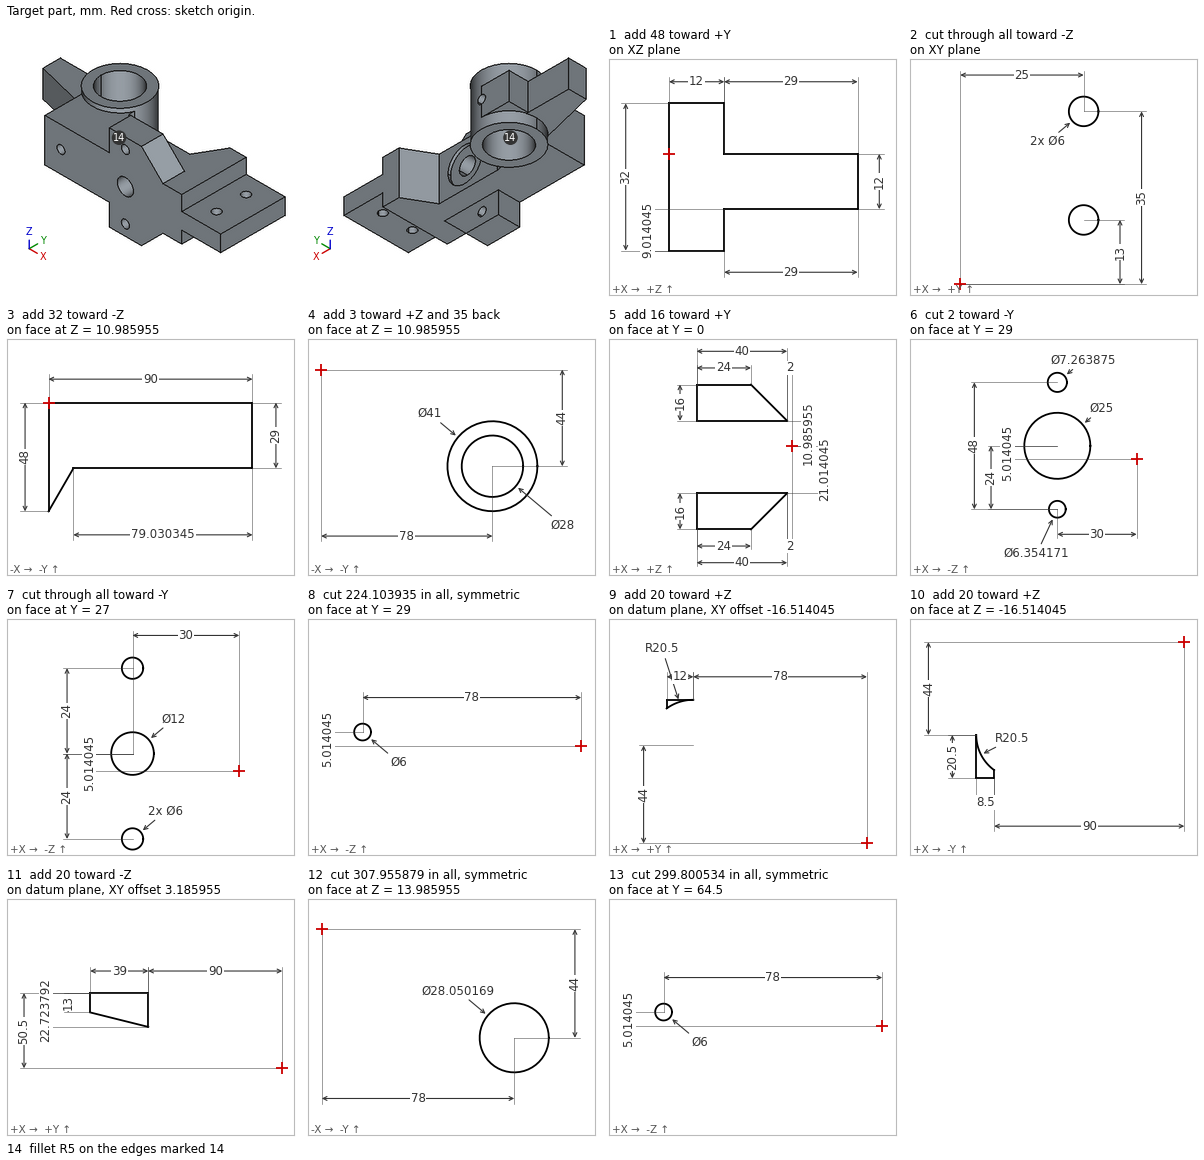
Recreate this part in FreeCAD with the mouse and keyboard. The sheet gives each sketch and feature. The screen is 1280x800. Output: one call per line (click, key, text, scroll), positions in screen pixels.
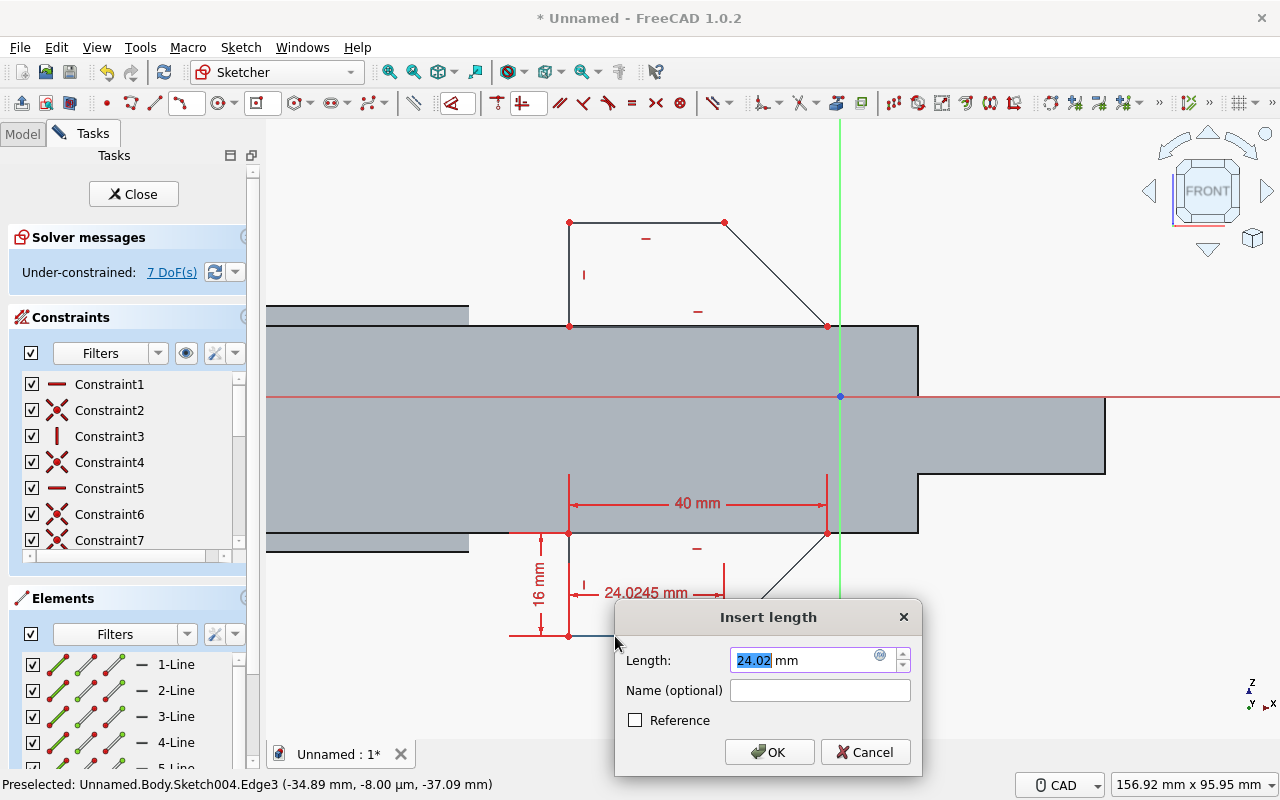
text(24)
key(Return)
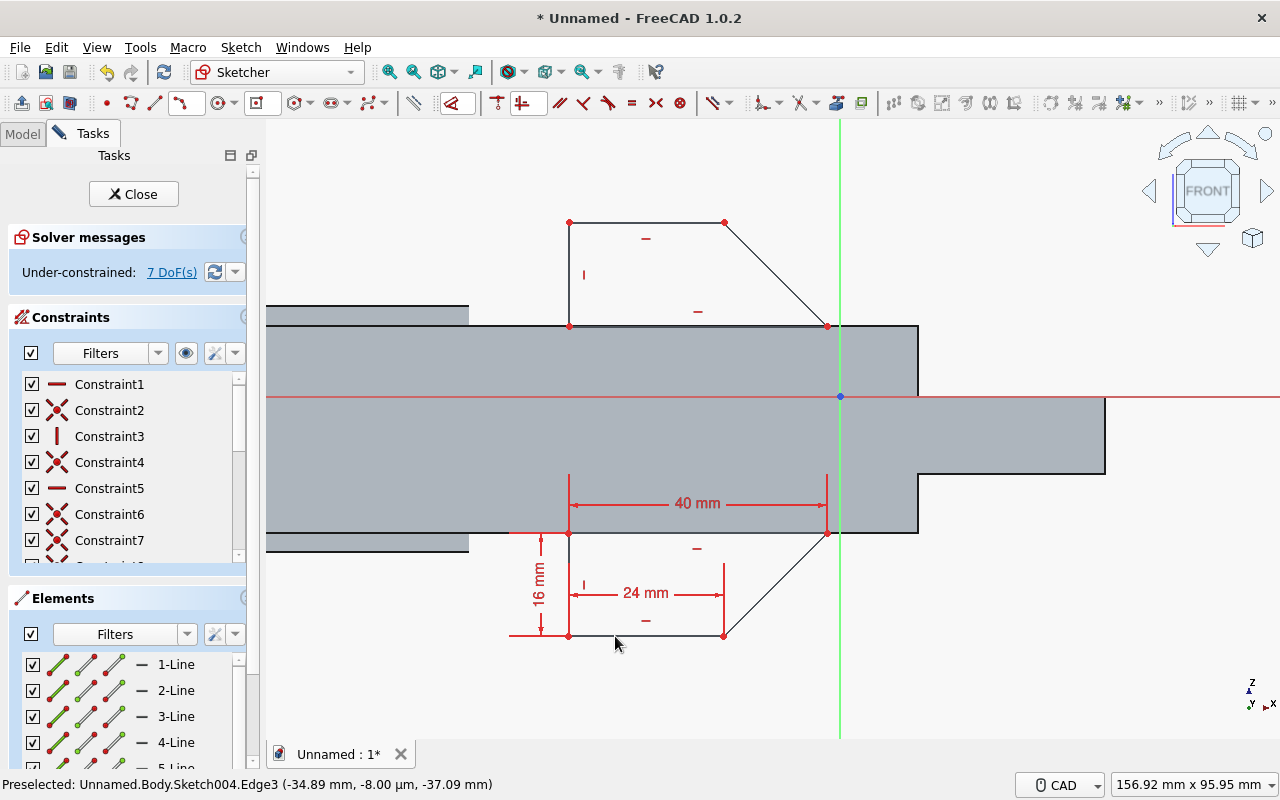
click(677, 223)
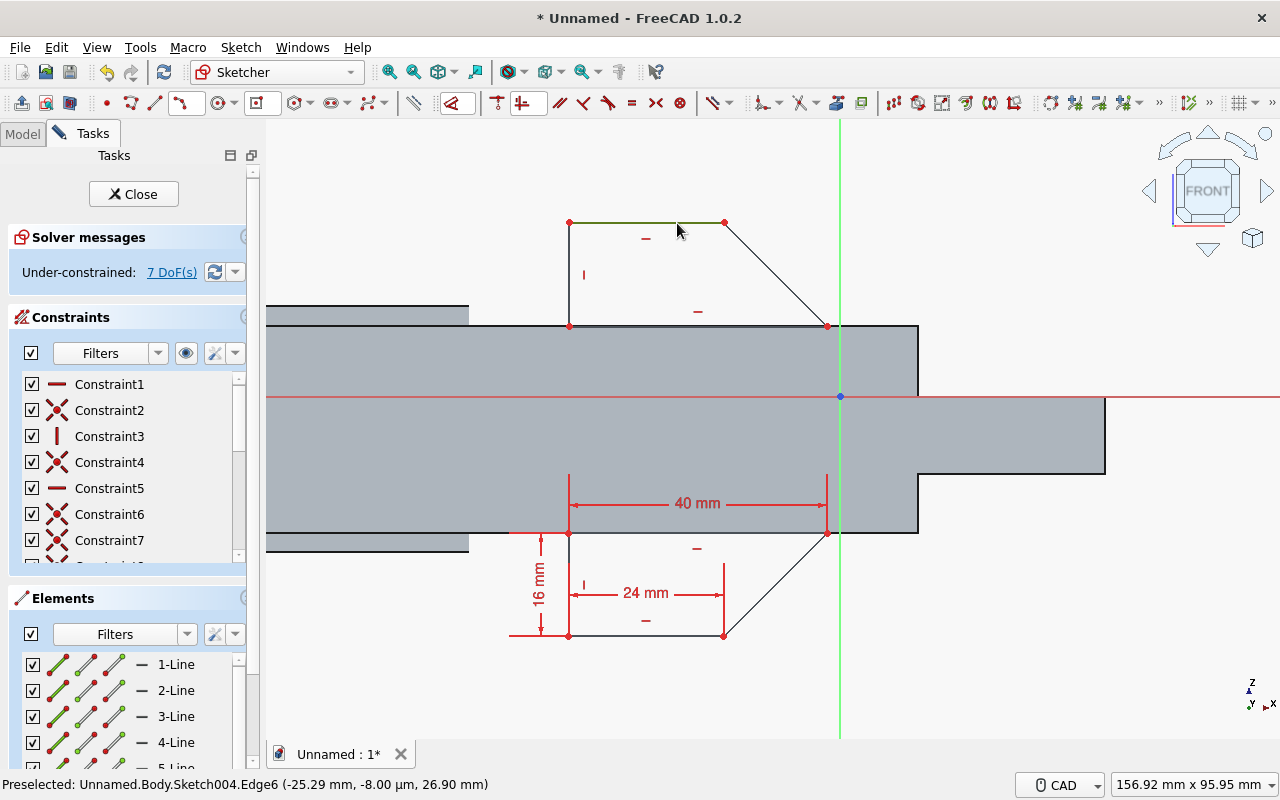
key(l)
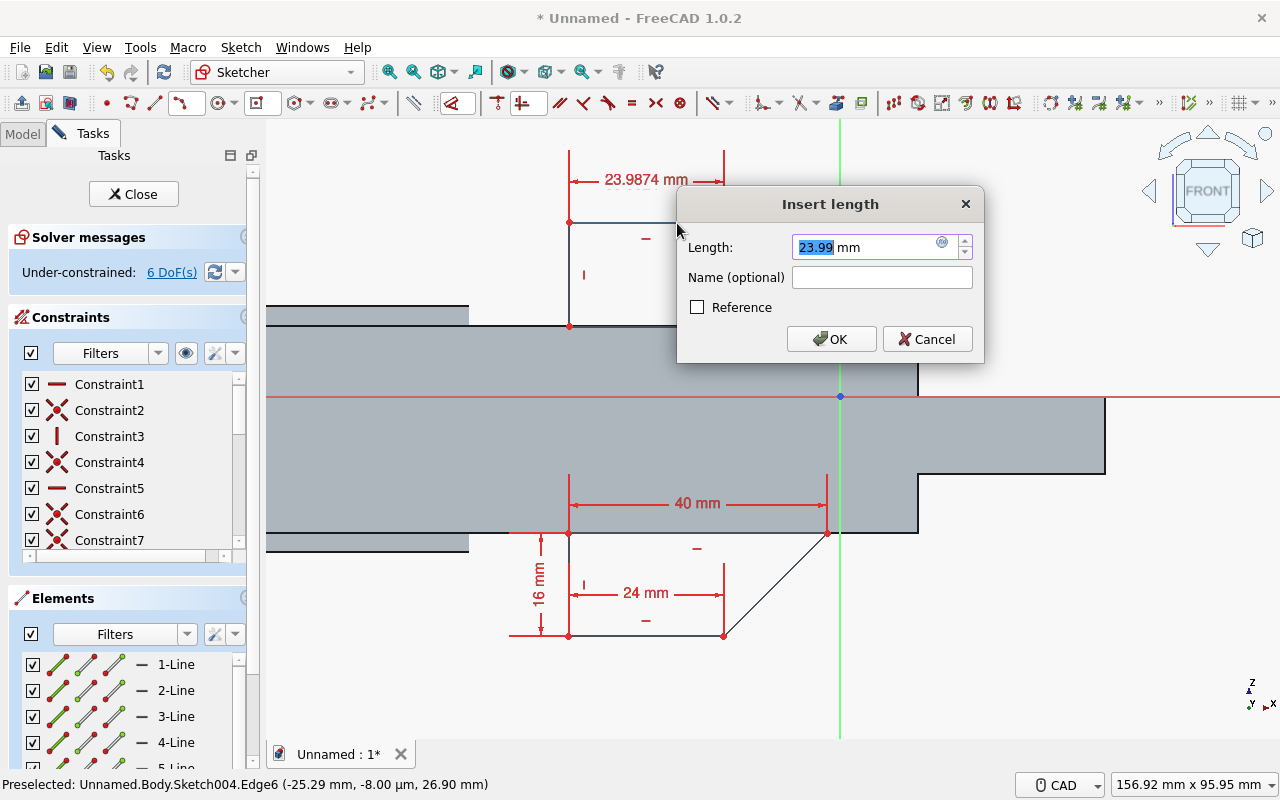
text(24)
key(Return)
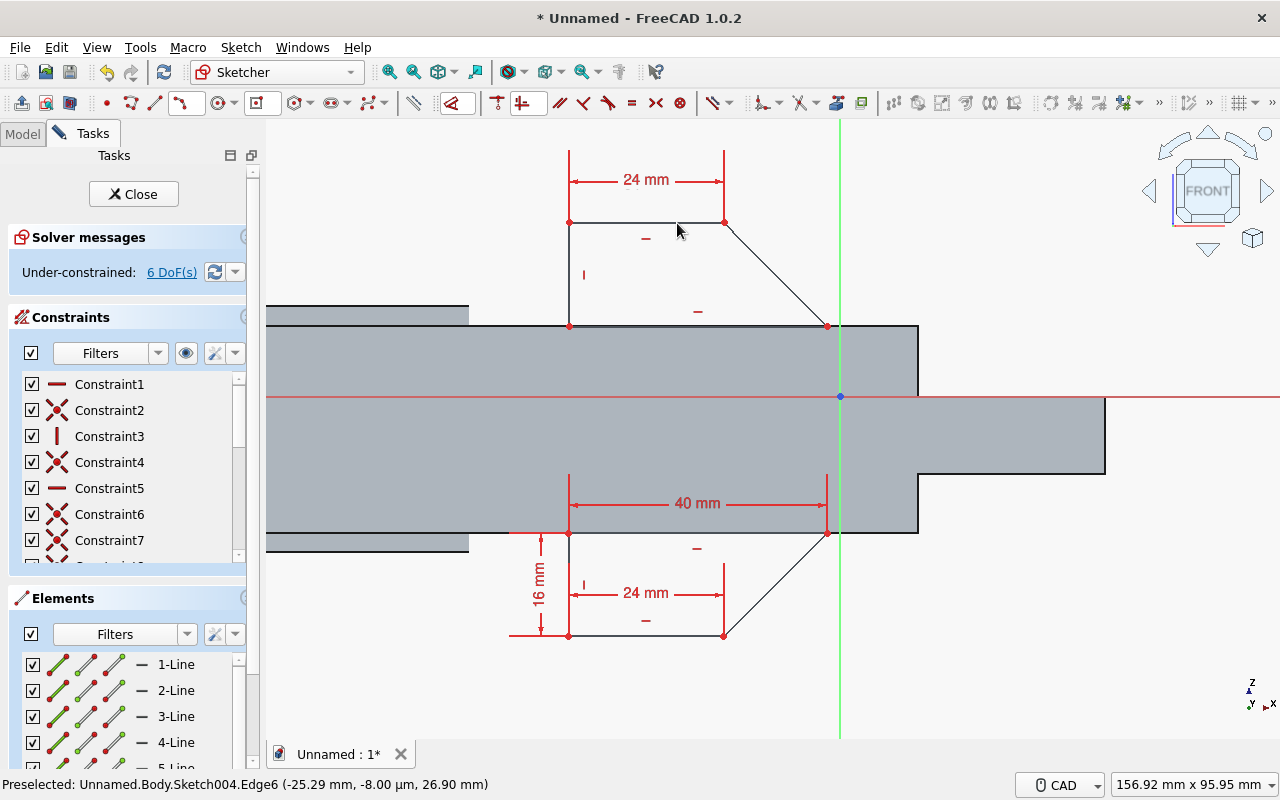
click(569, 254)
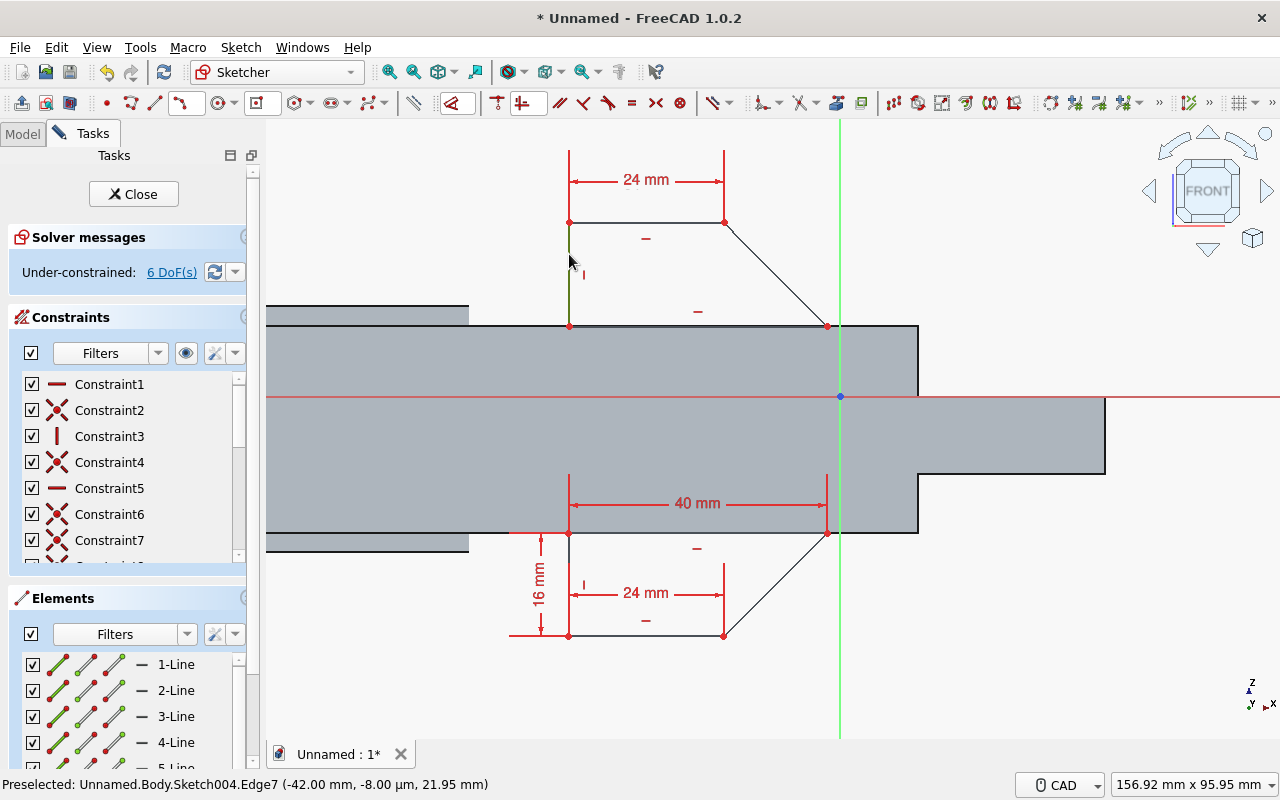
click(470, 104)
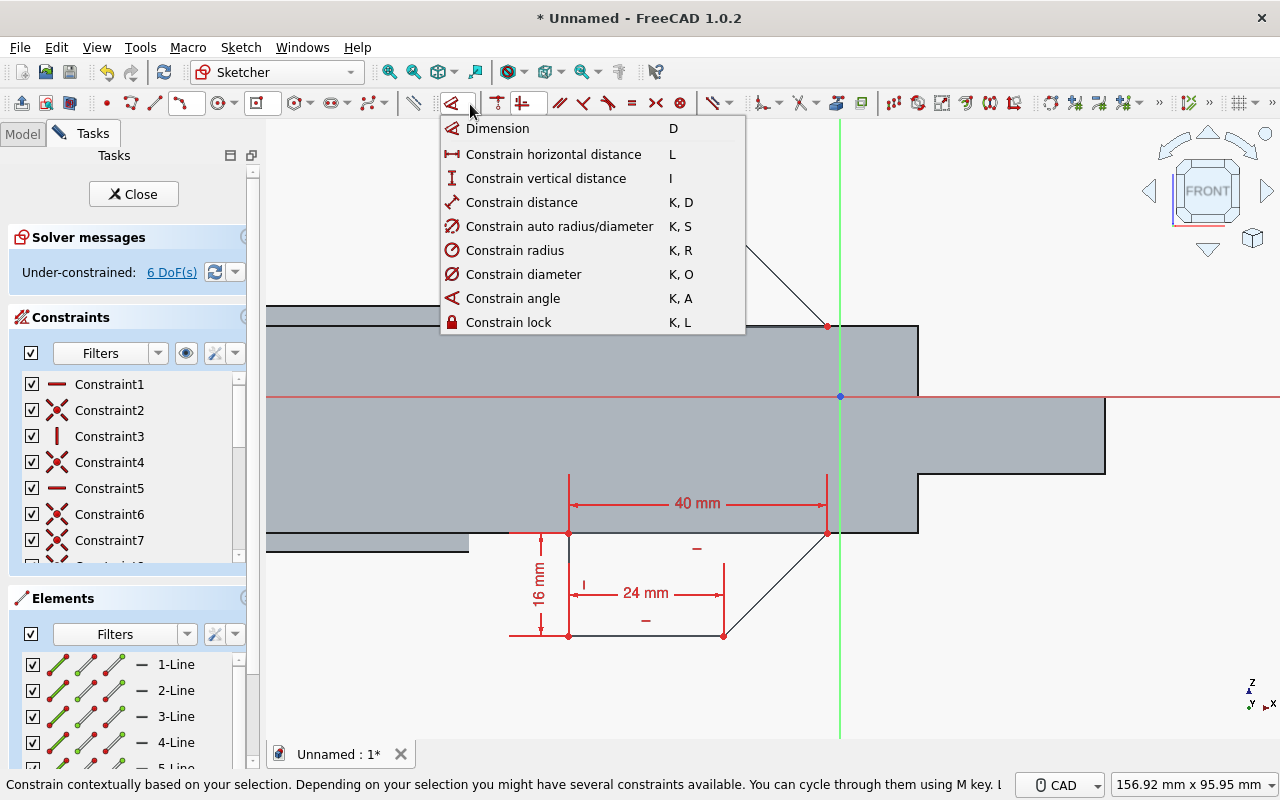
click(593, 178)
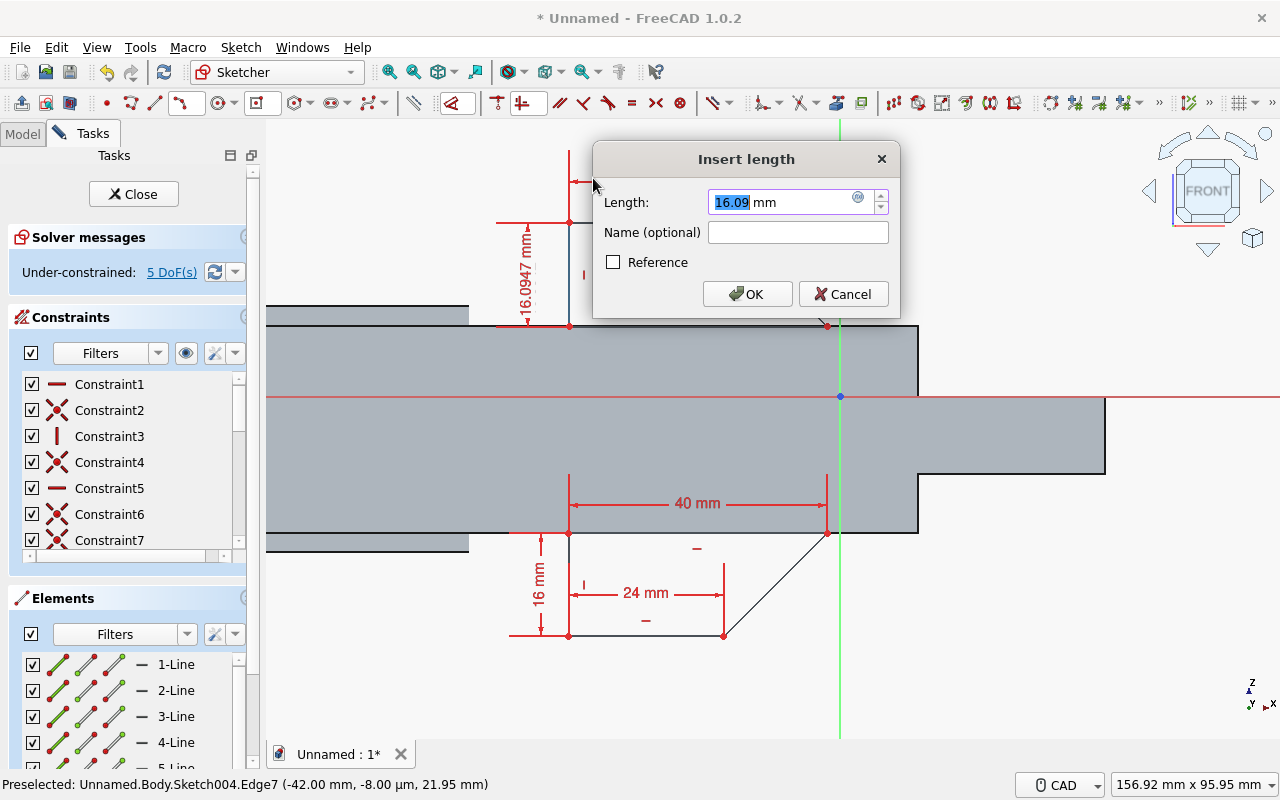
text(16)
key(Return)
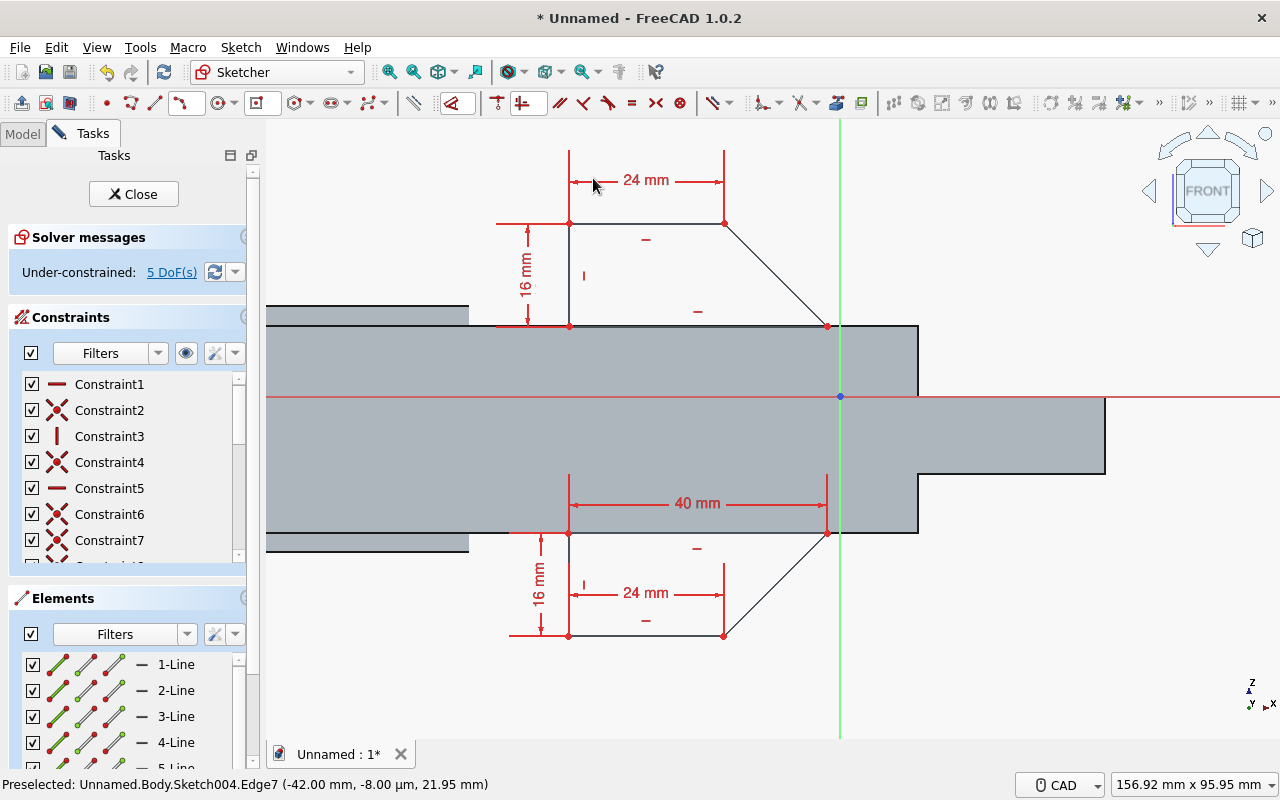
click(646, 327)